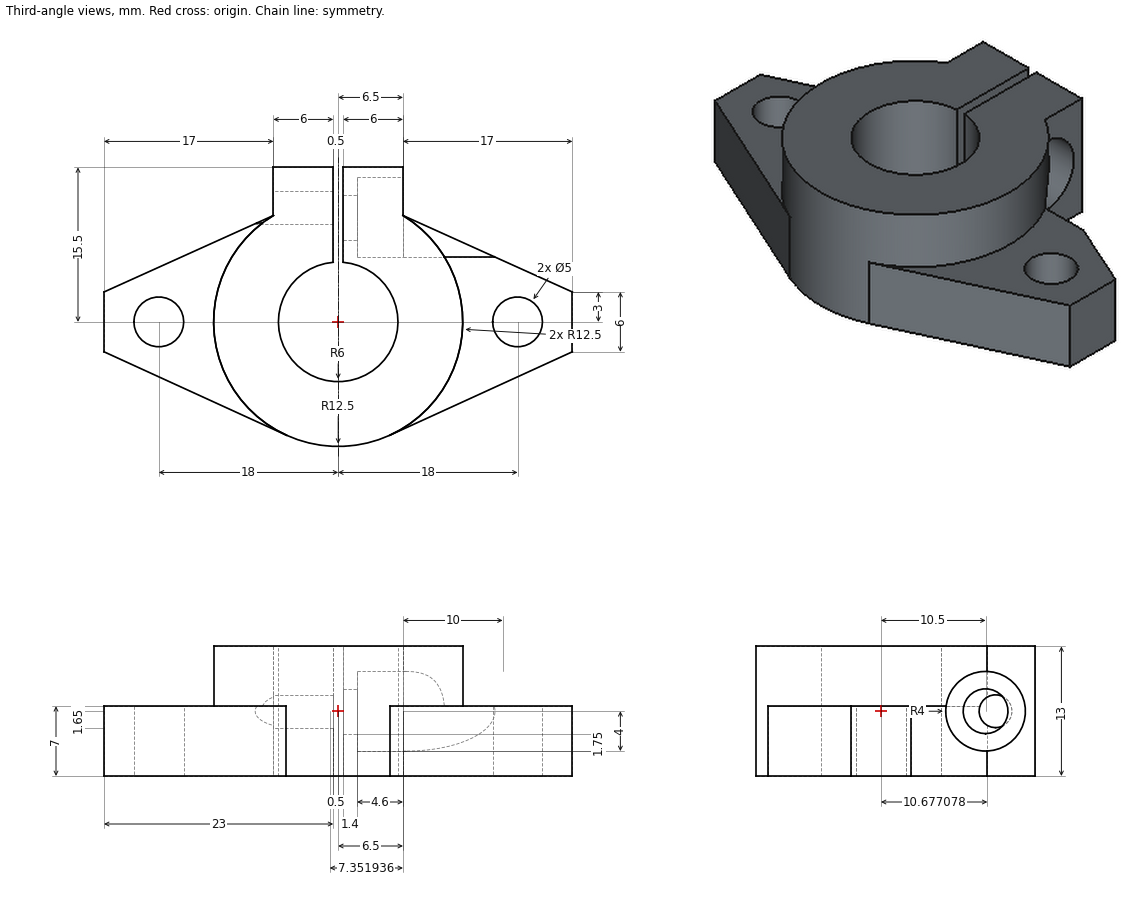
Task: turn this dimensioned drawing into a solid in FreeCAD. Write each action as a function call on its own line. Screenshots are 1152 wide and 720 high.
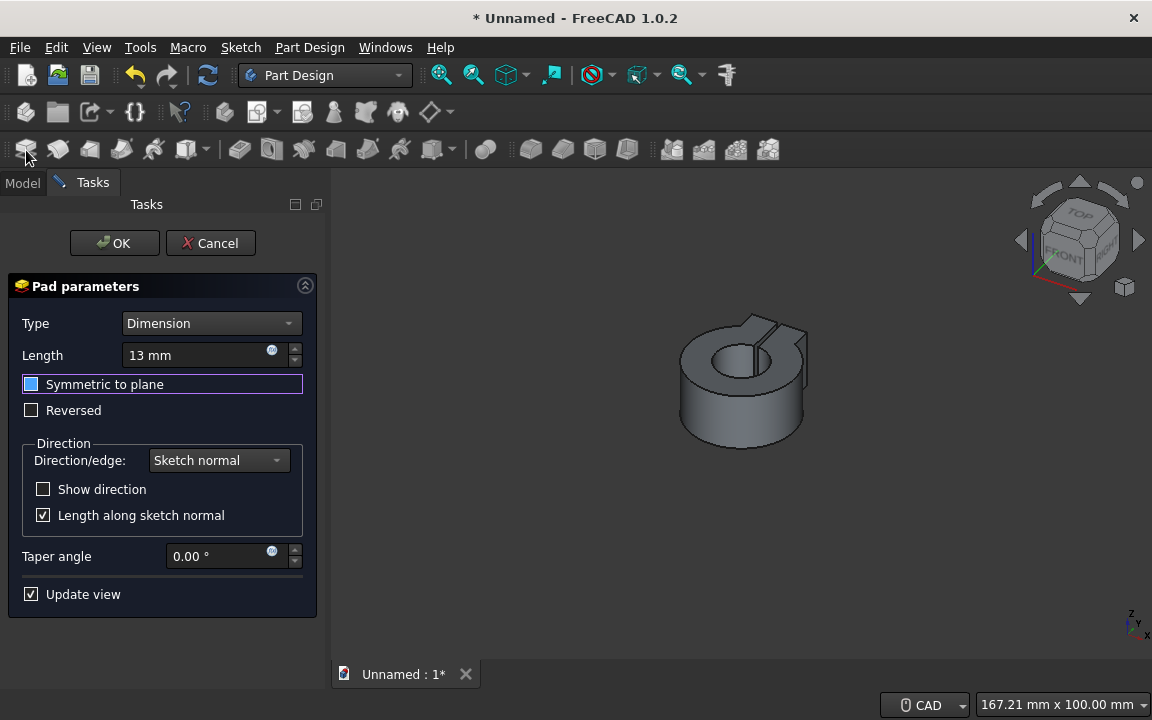
click(30, 384)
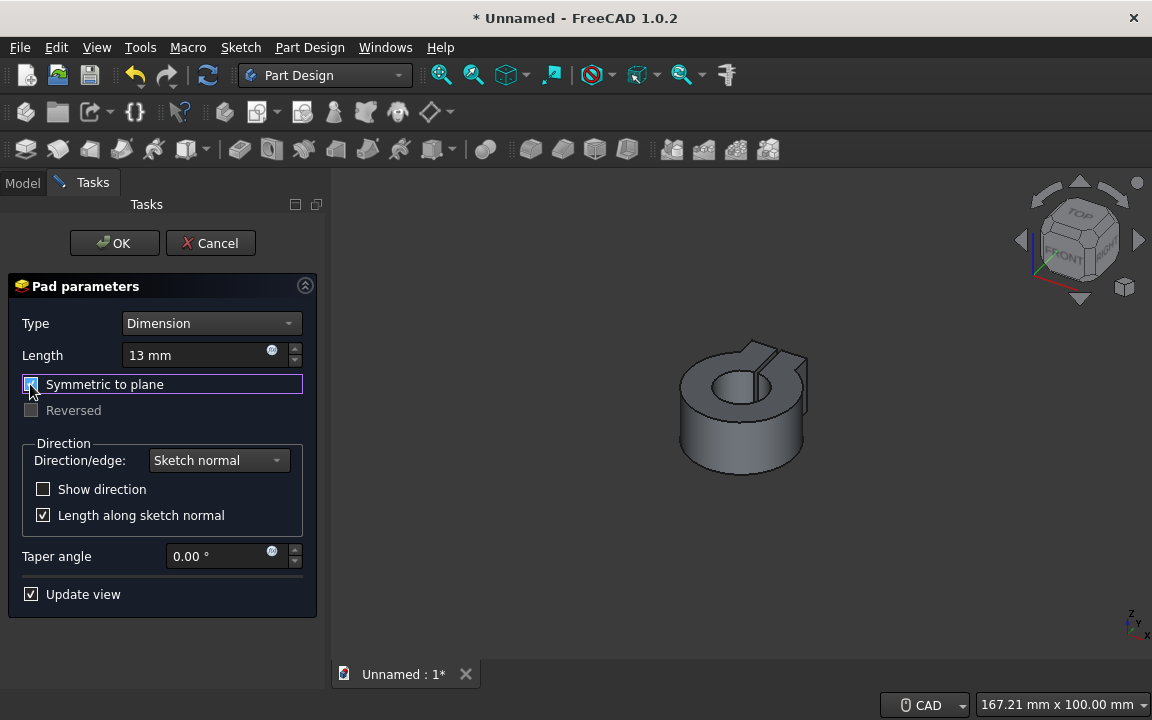
click(115, 243)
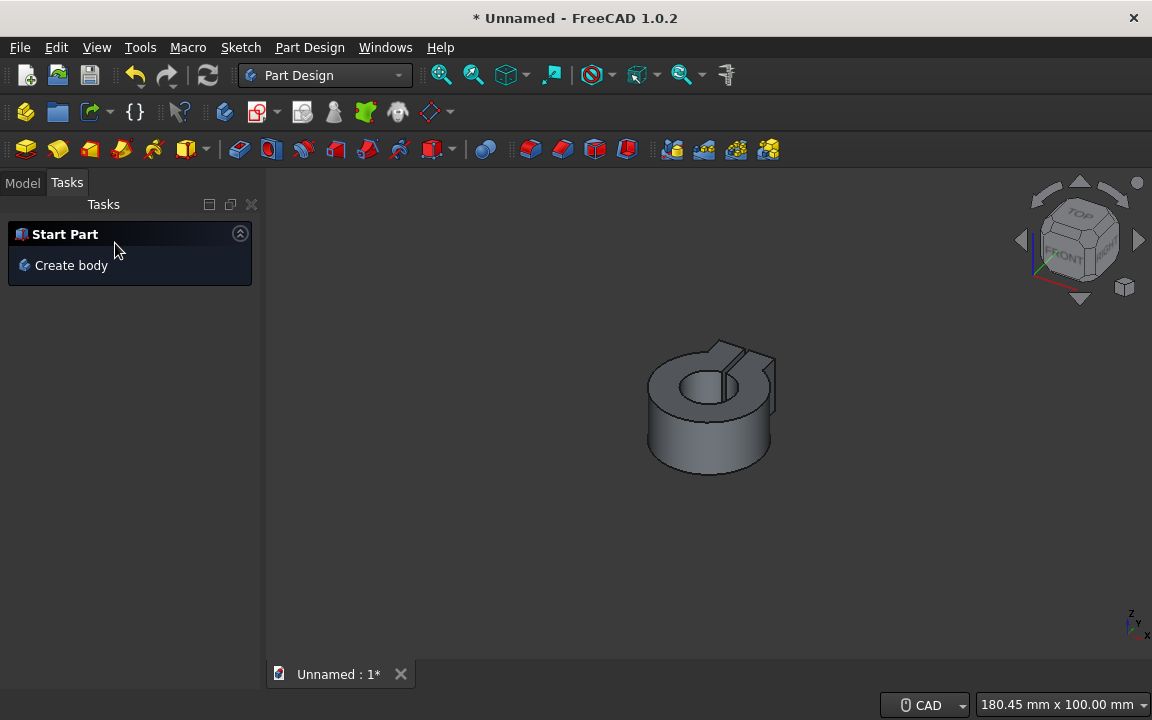
click(442, 76)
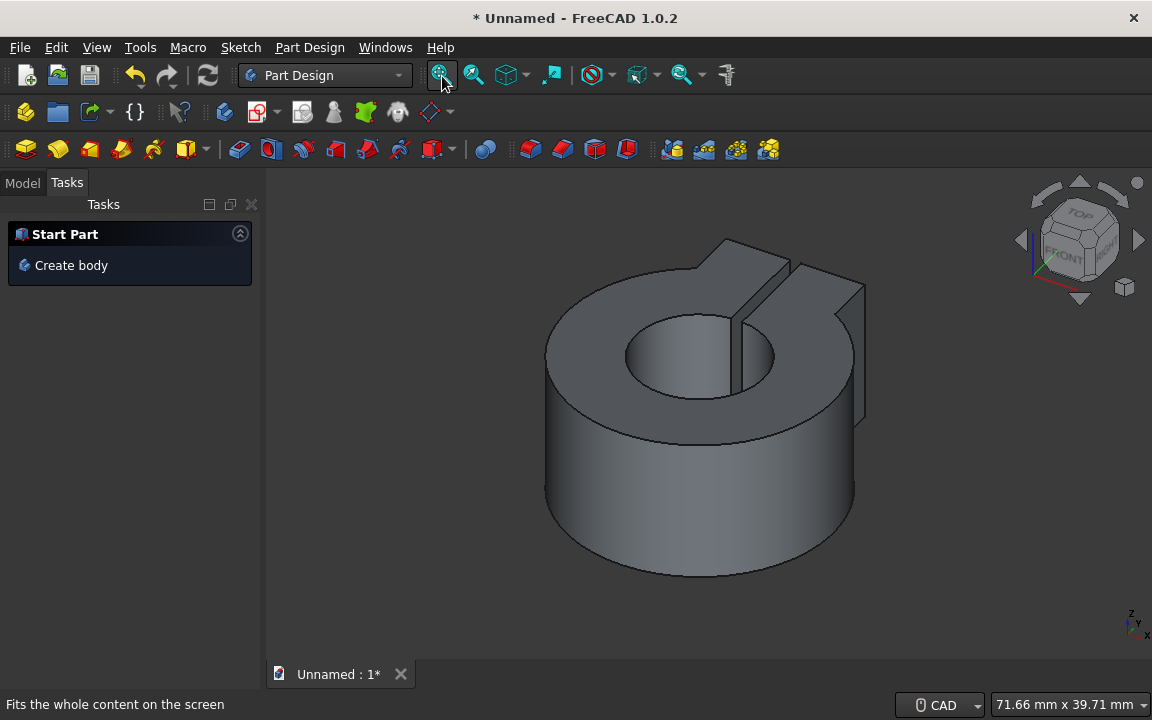
click(23, 182)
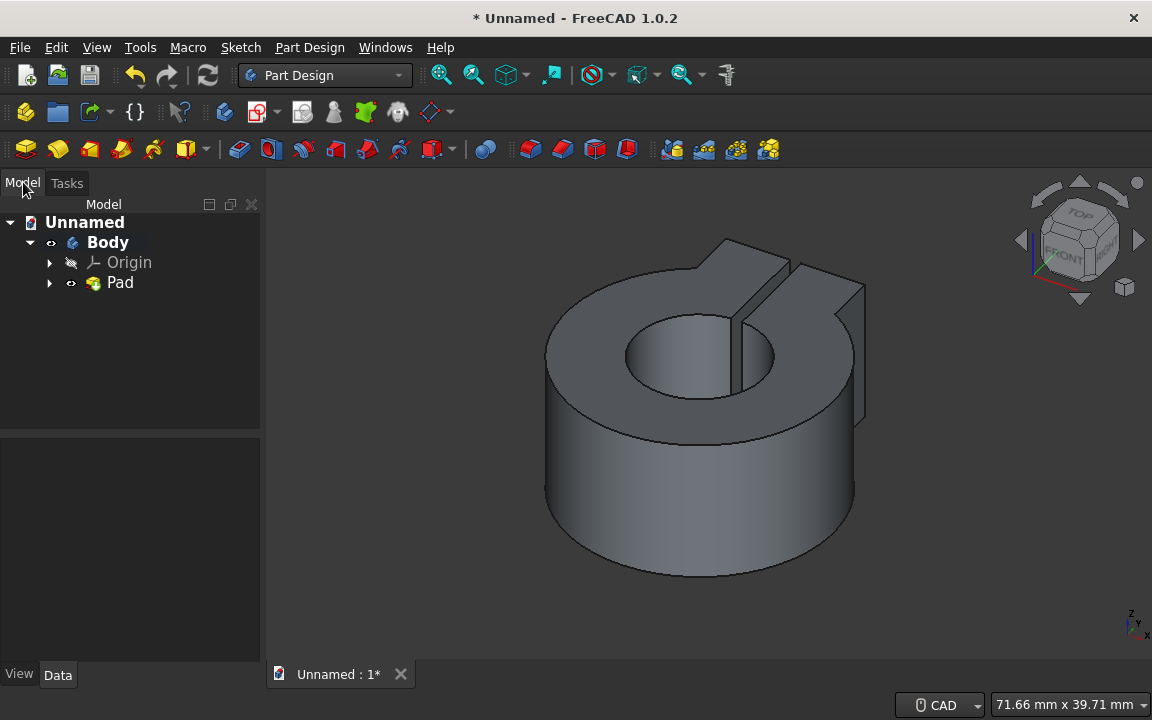
click(50, 263)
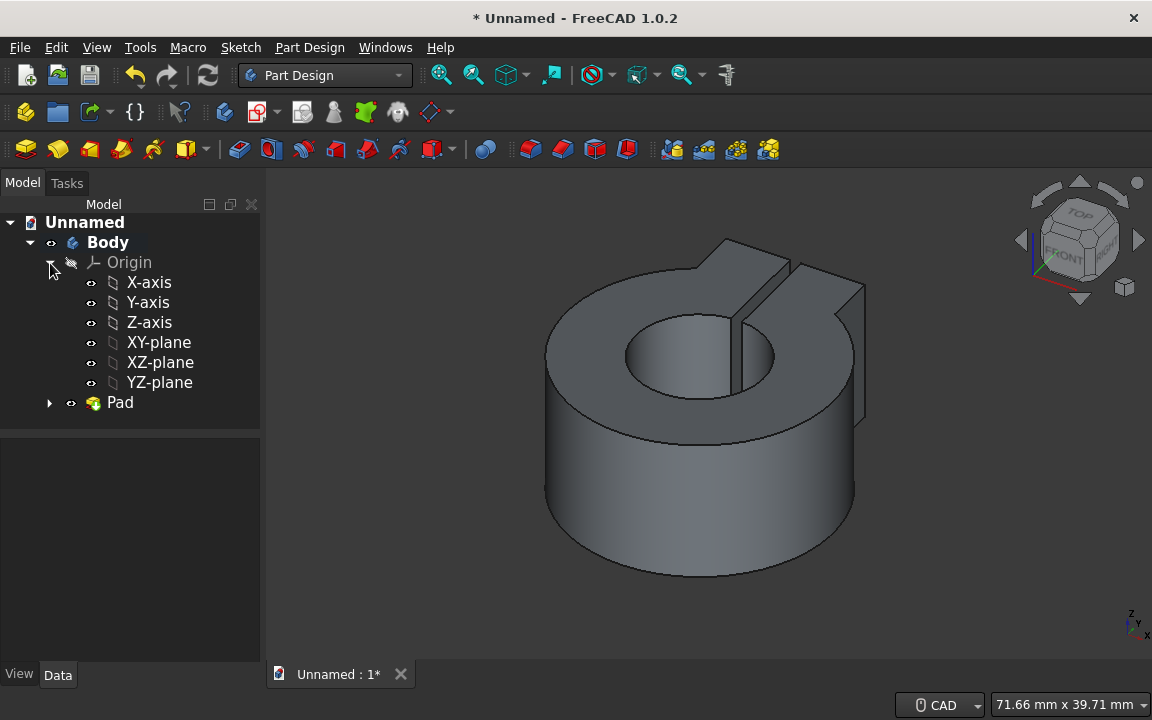
click(136, 343)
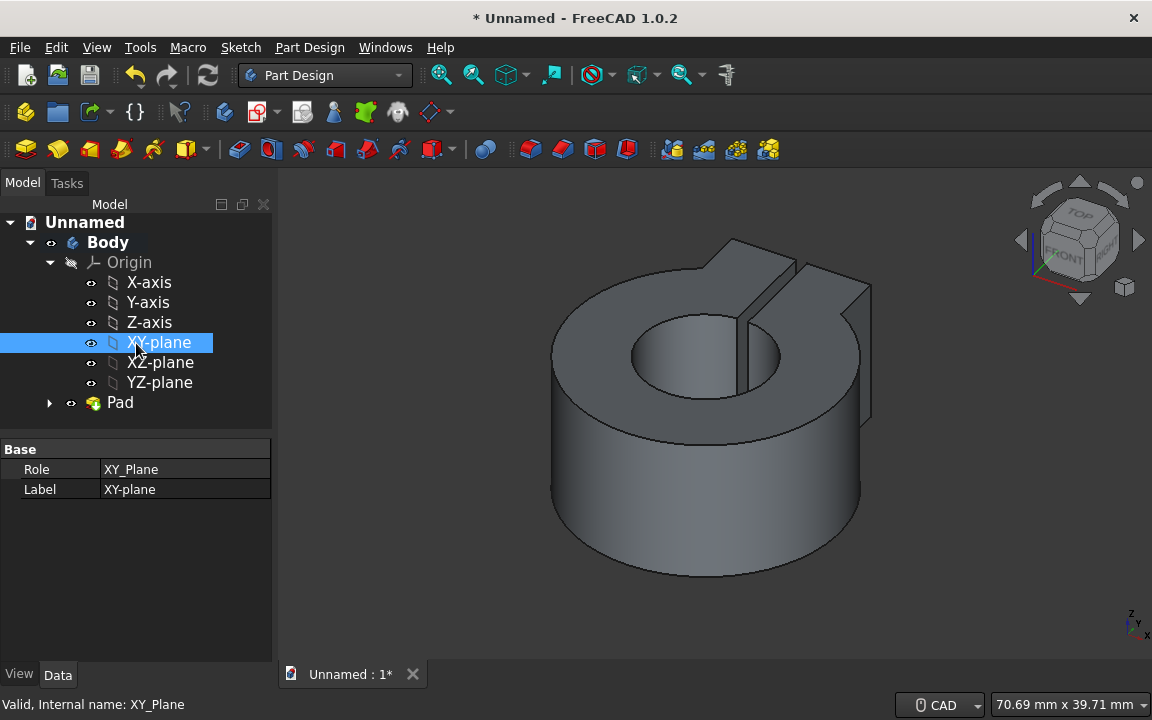
click(430, 112)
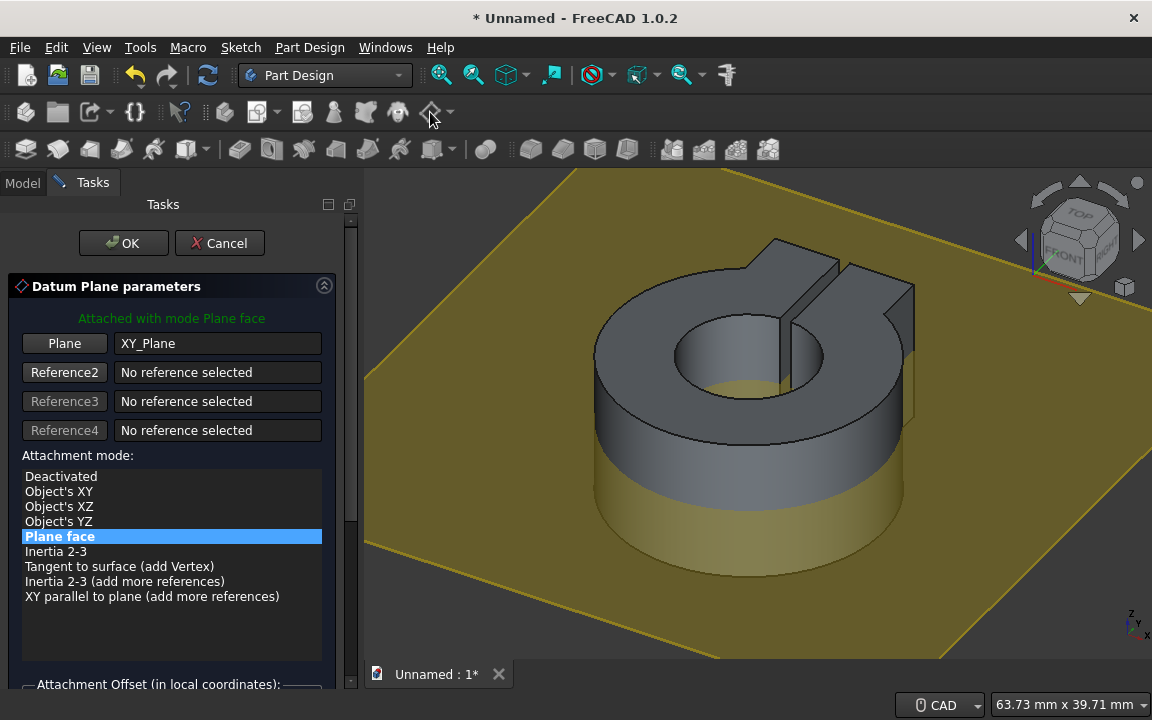
scroll(351, 451, down, 3)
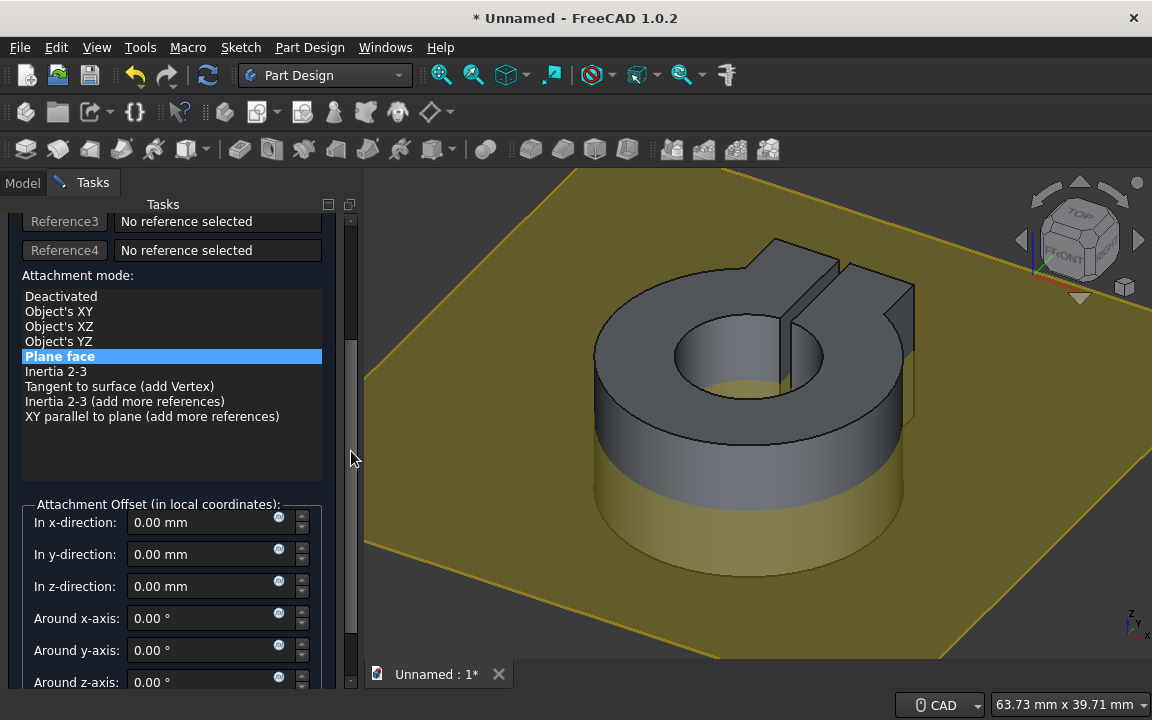
triple_click(210, 586)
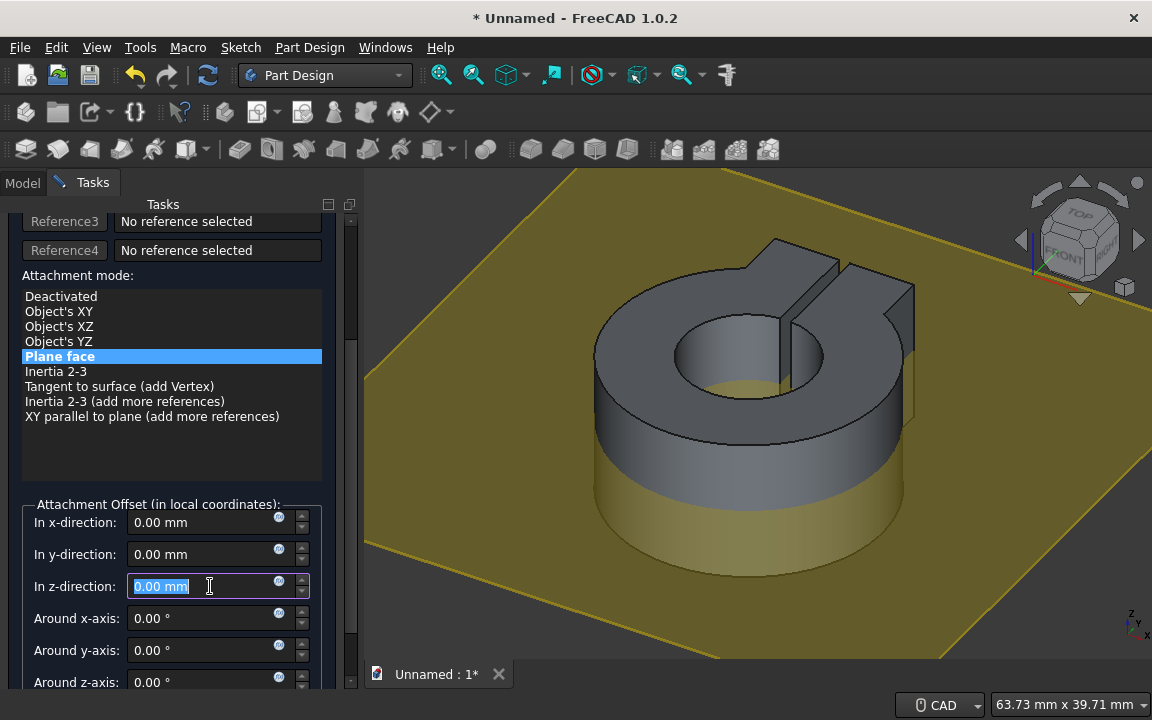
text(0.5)
key(Tab)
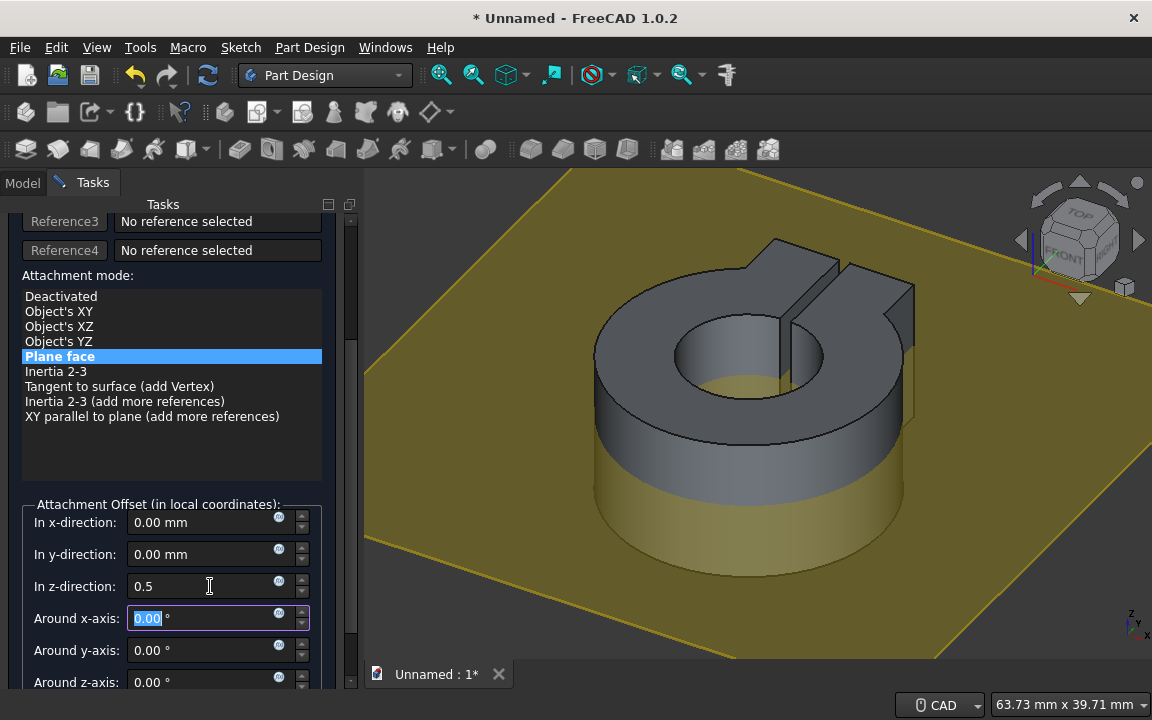
scroll(351, 451, up, 4)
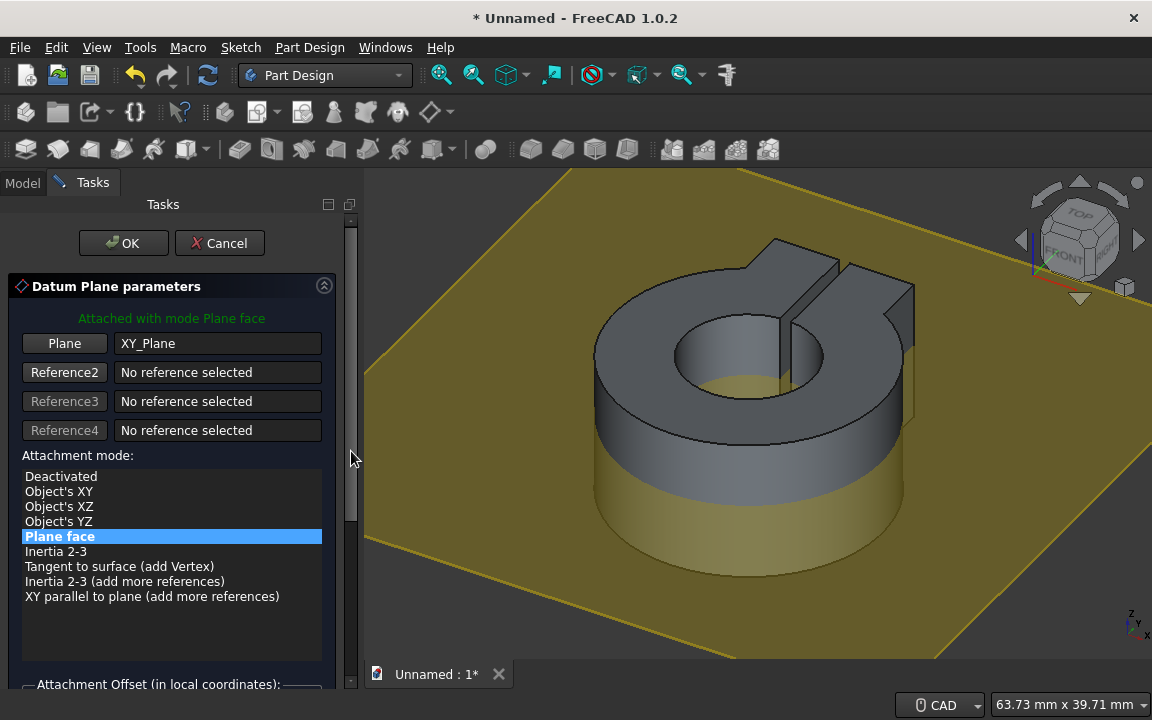
click(124, 243)